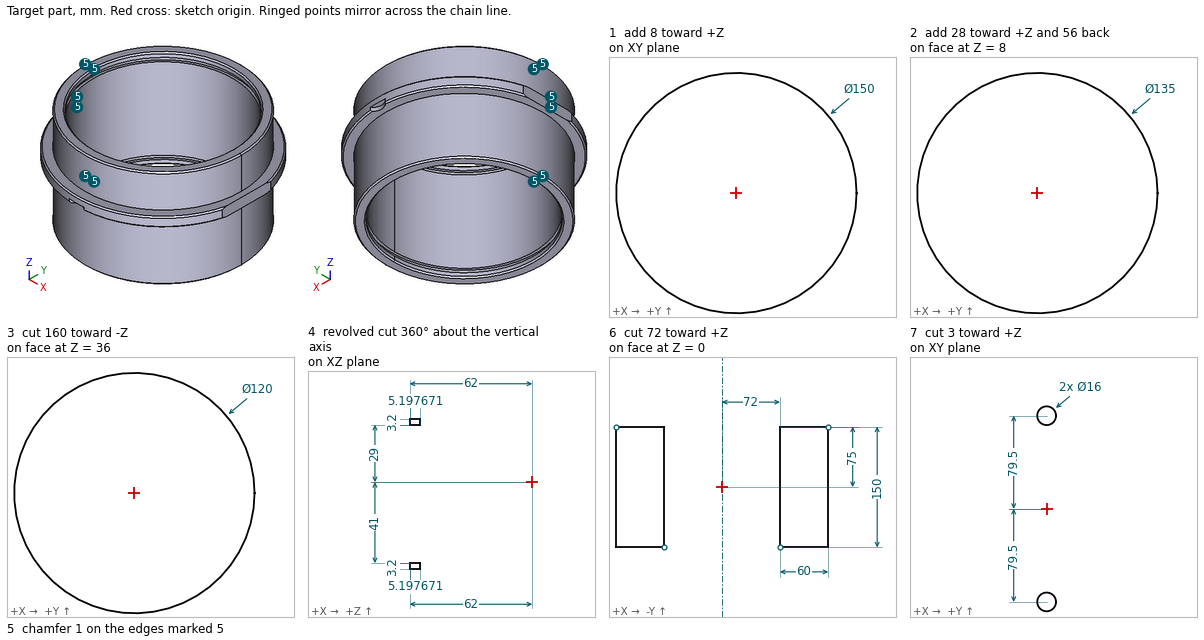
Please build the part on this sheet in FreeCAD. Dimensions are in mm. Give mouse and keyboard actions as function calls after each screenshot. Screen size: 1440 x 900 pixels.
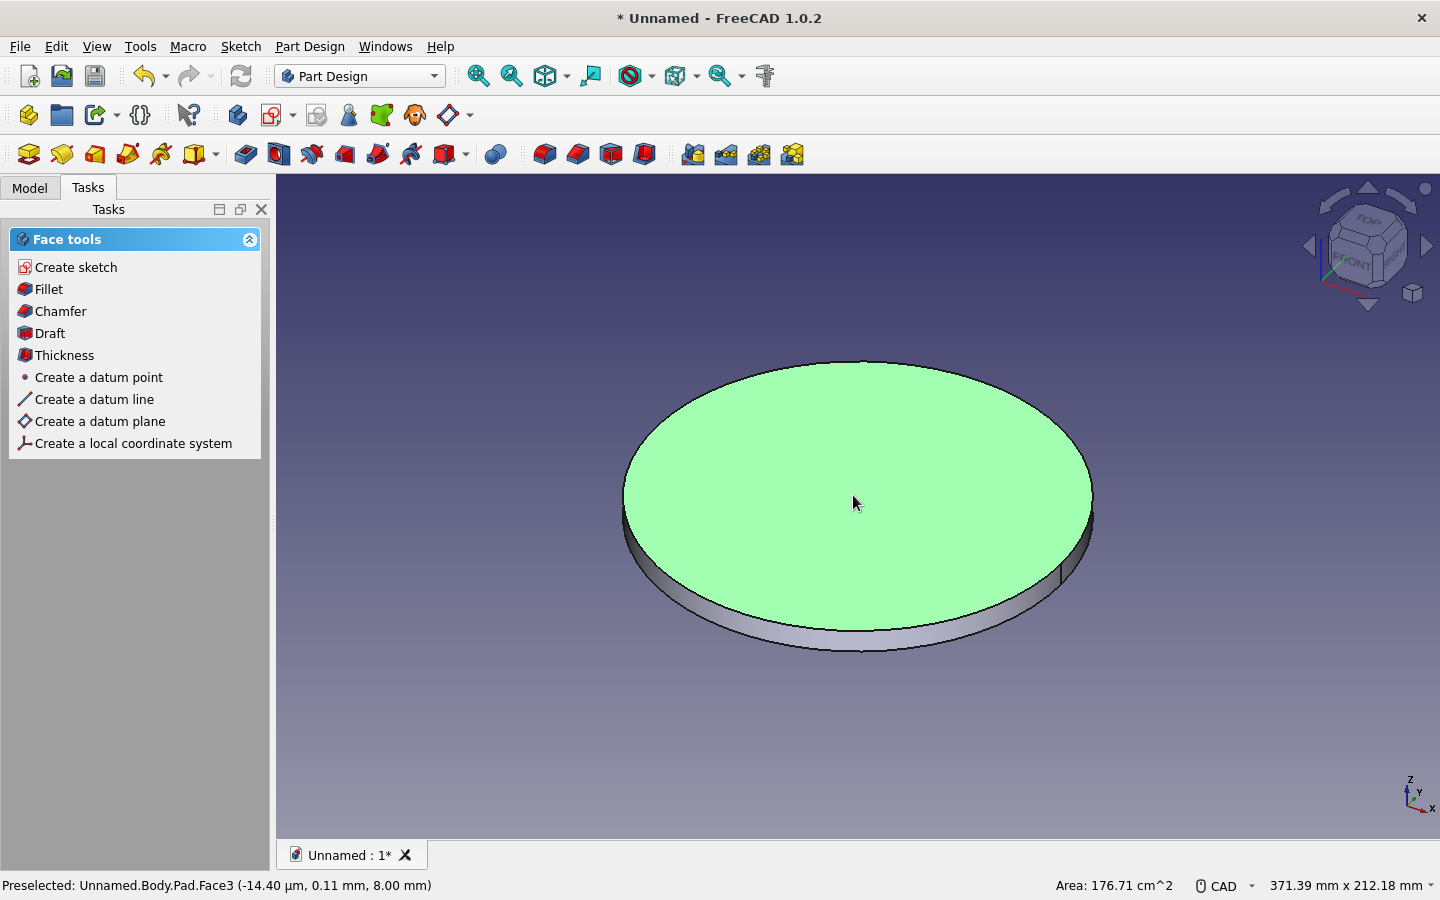
click(270, 116)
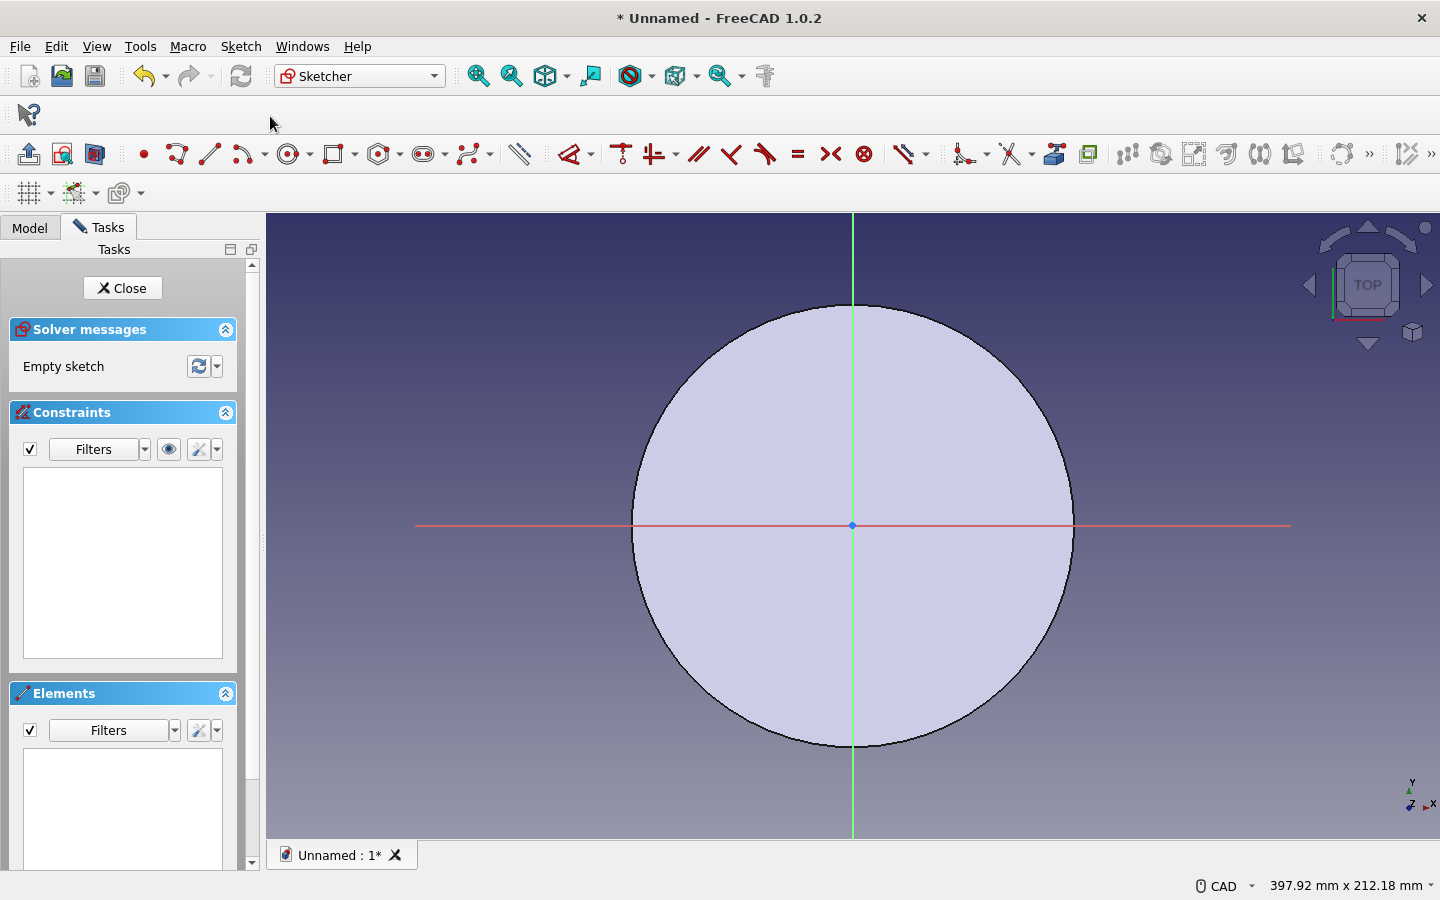
key(g)
key(c)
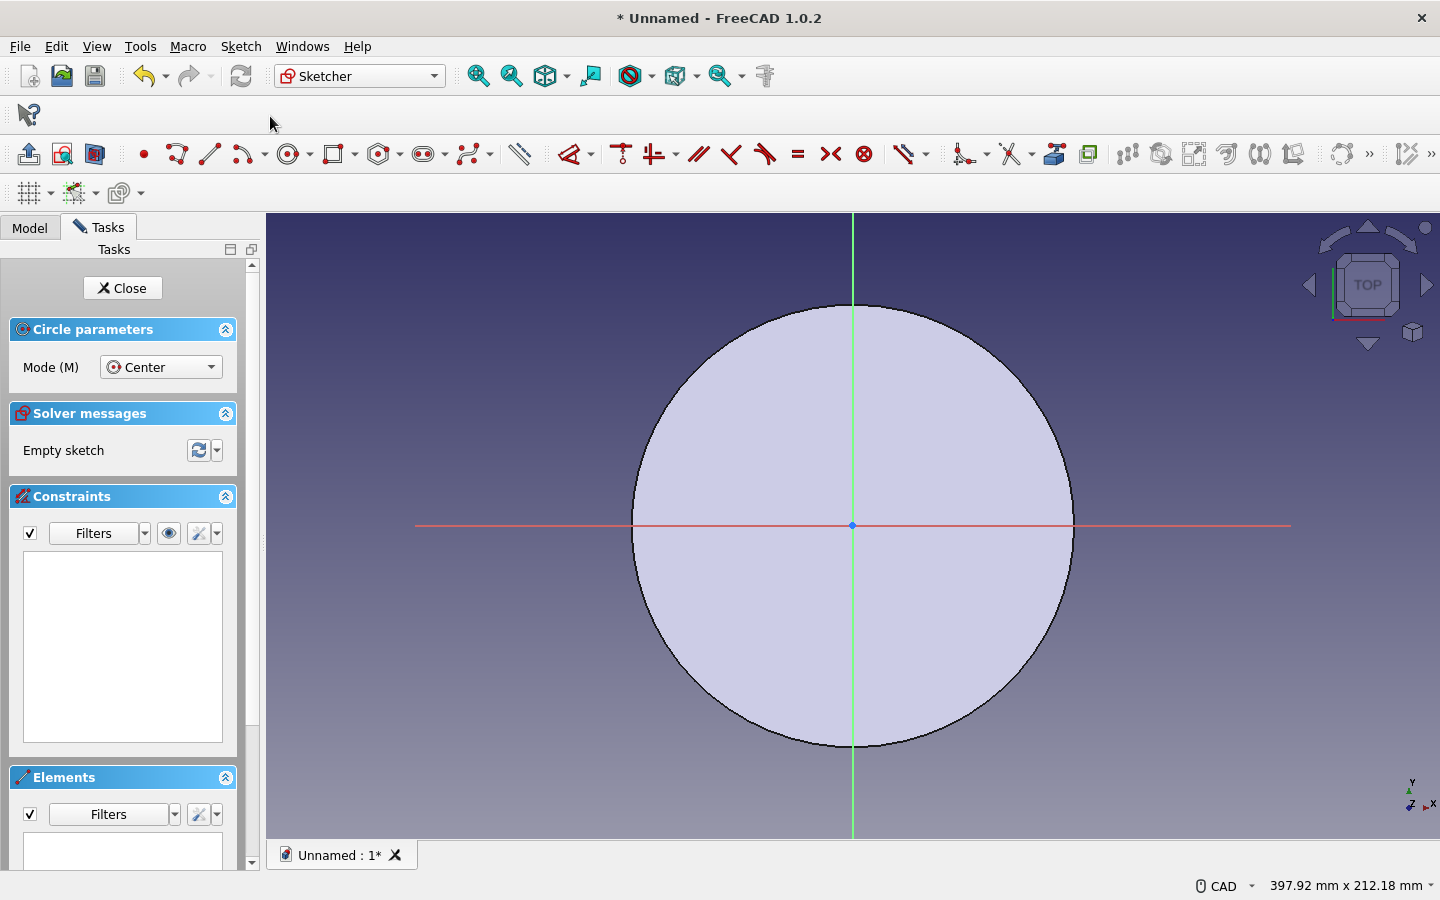
click(853, 526)
click(994, 385)
key(Escape)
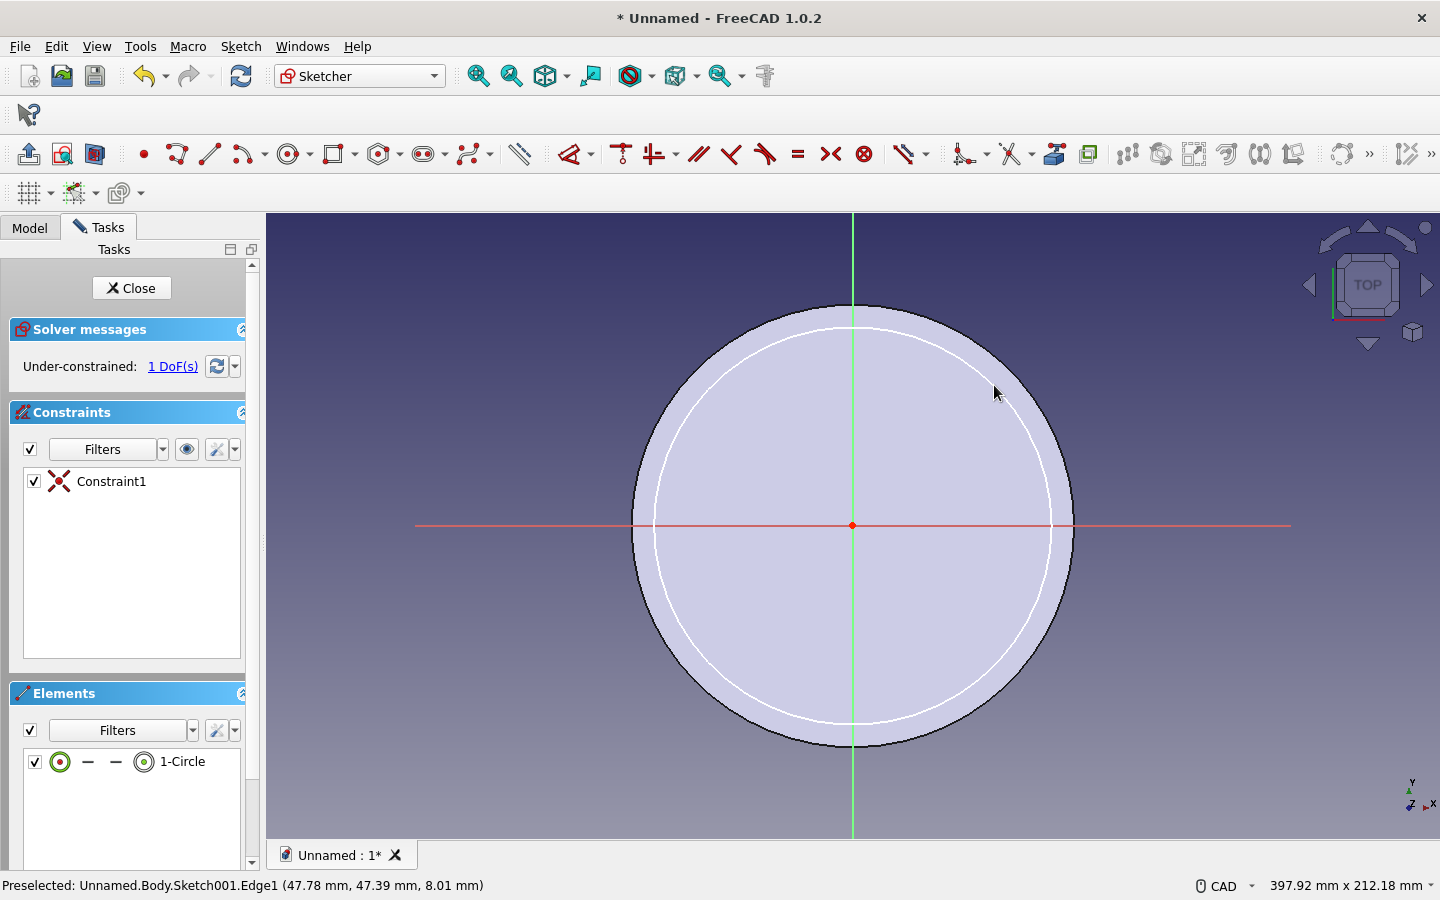
key(d)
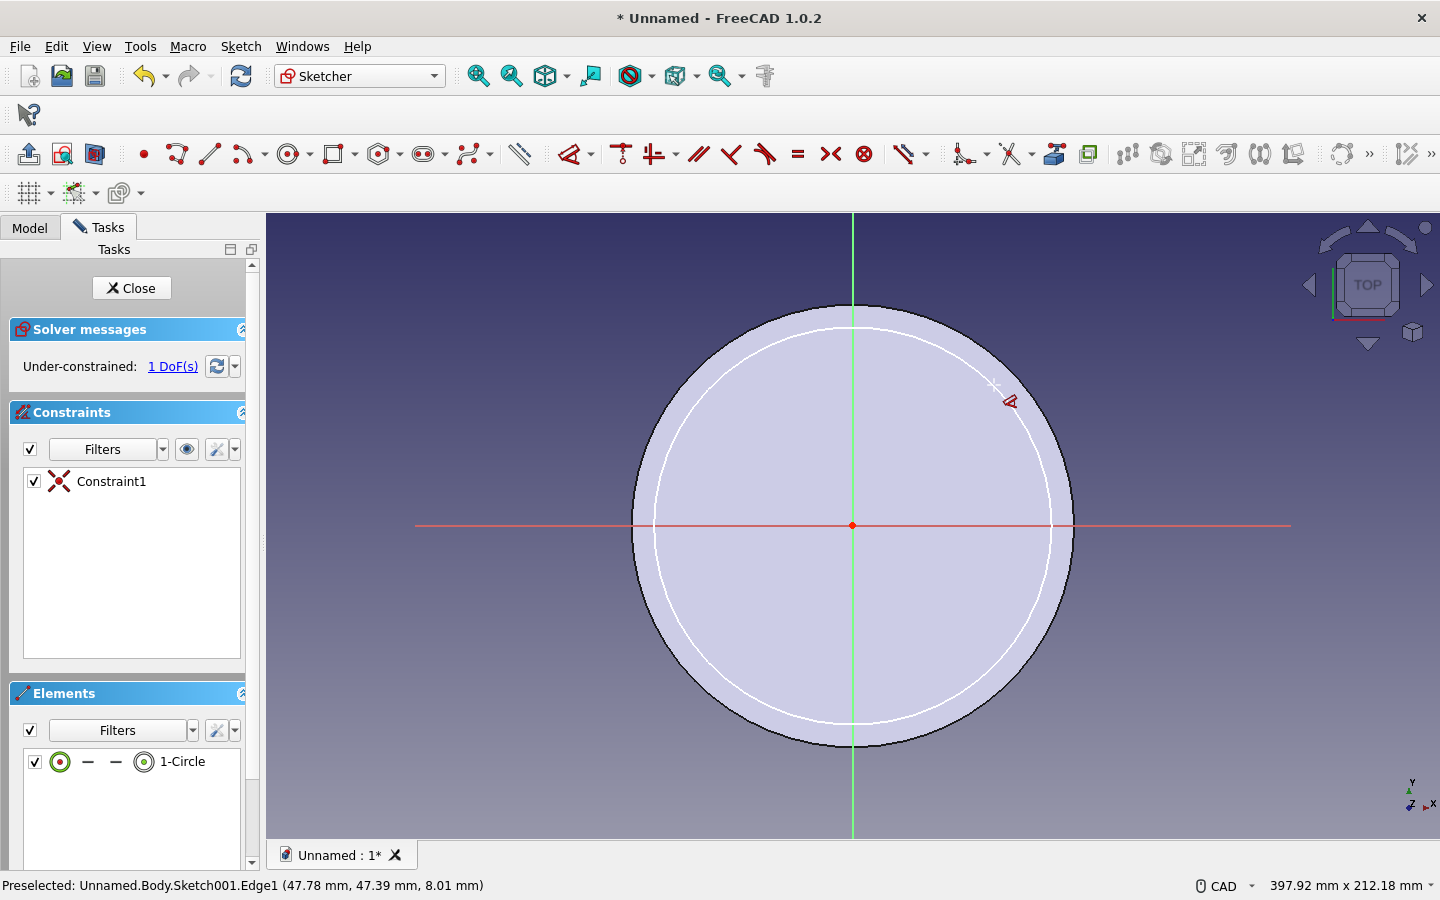
click(993, 385)
click(1016, 362)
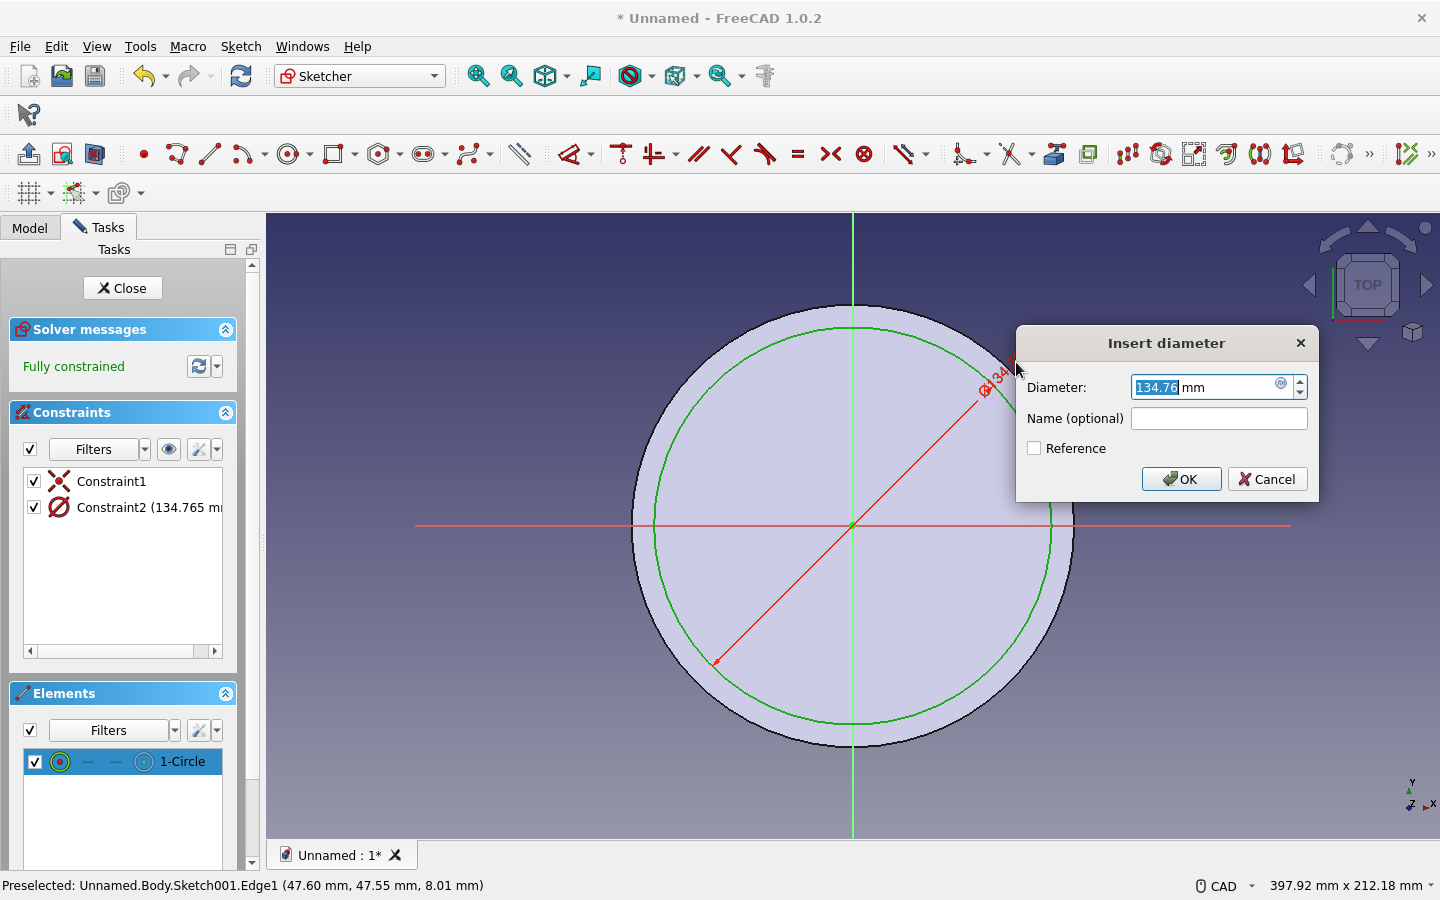
text(135)
key(Return)
key(Escape)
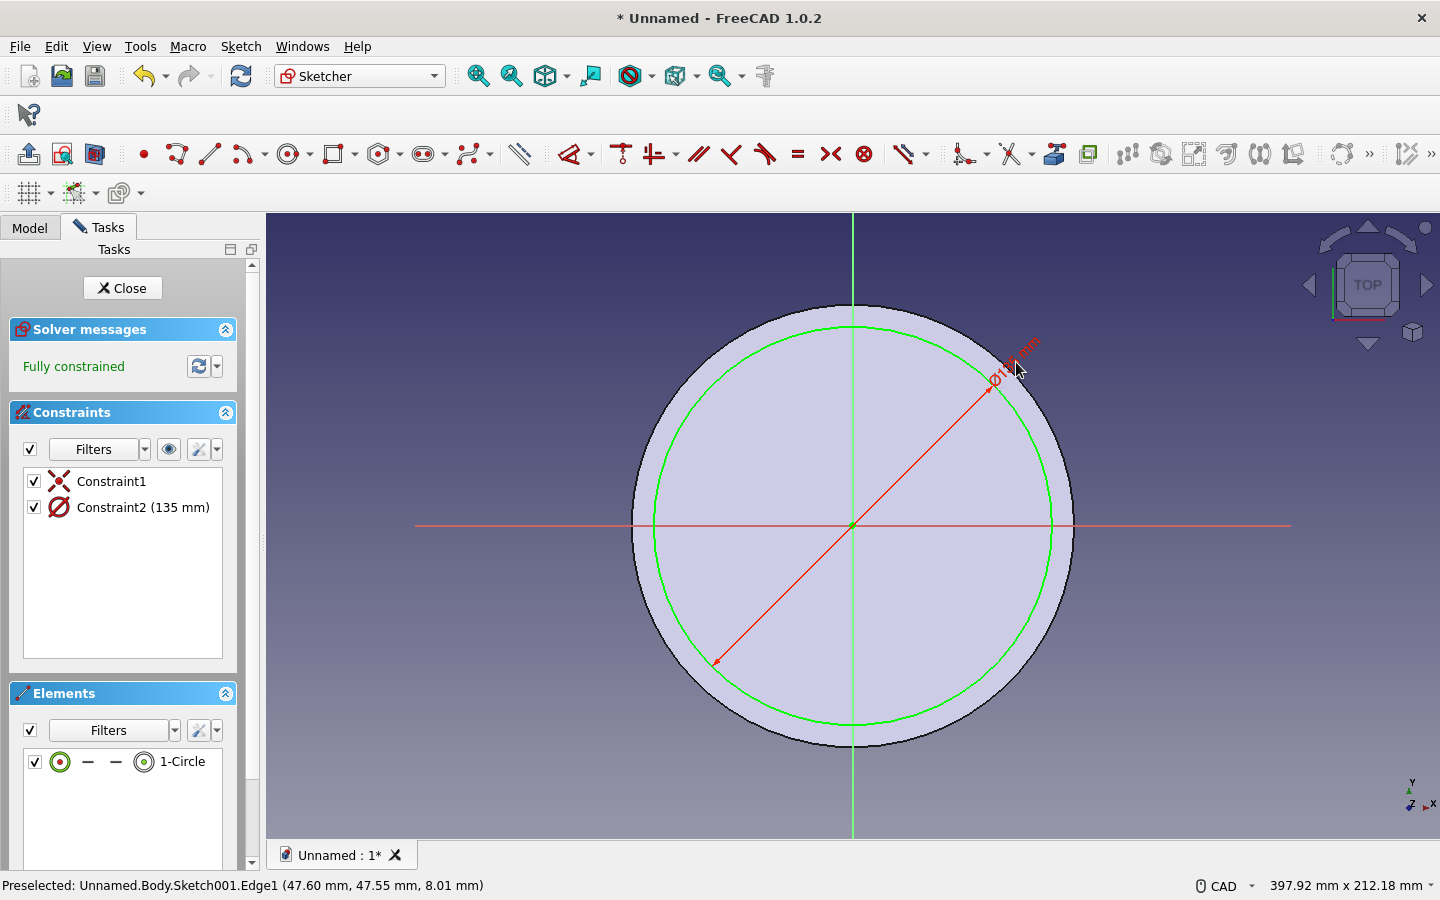
click(123, 288)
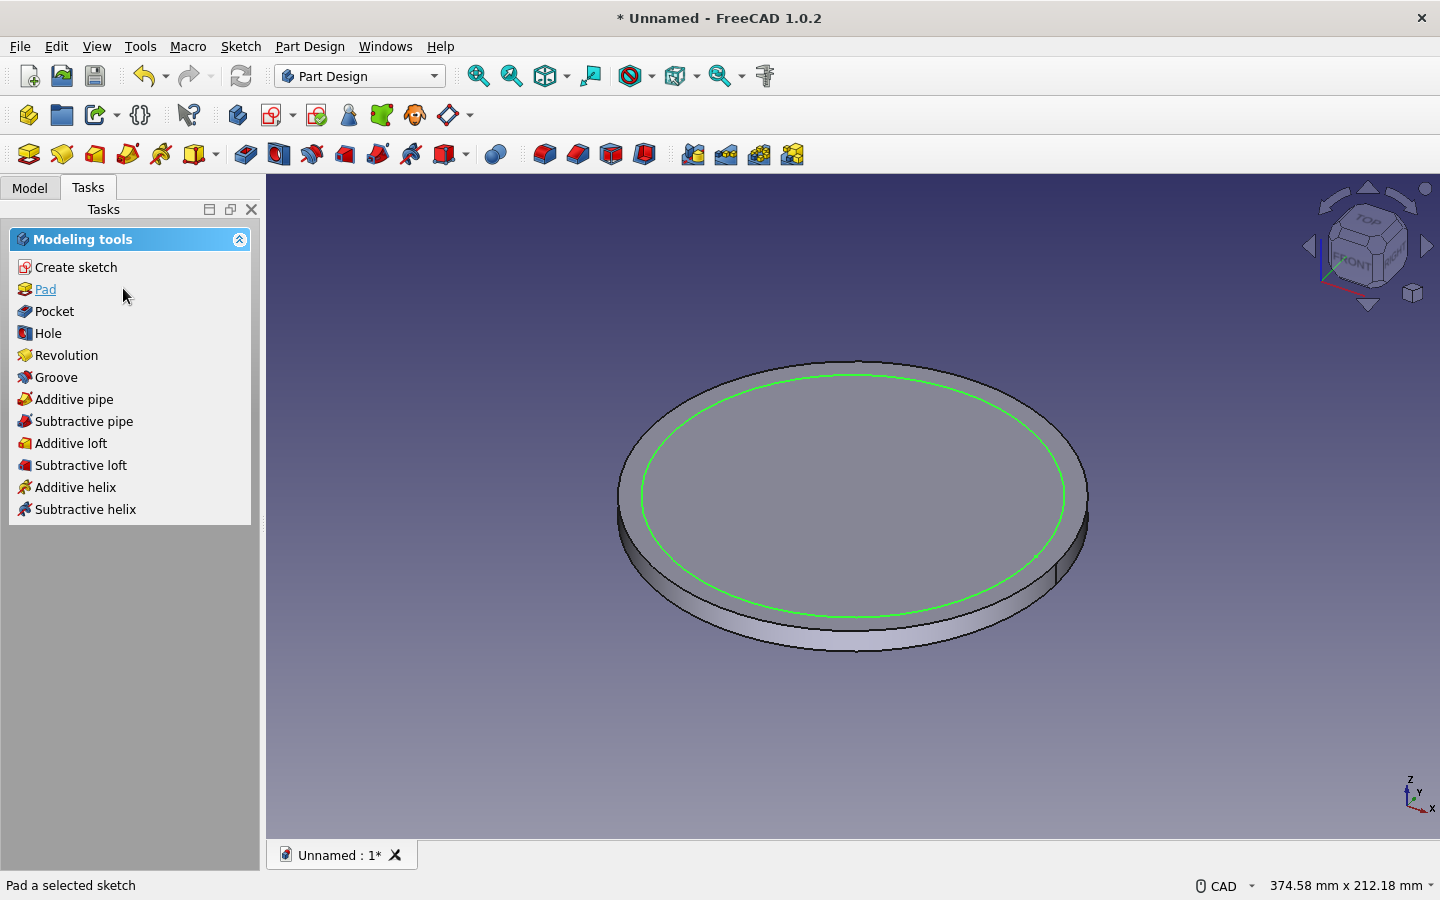
click(29, 154)